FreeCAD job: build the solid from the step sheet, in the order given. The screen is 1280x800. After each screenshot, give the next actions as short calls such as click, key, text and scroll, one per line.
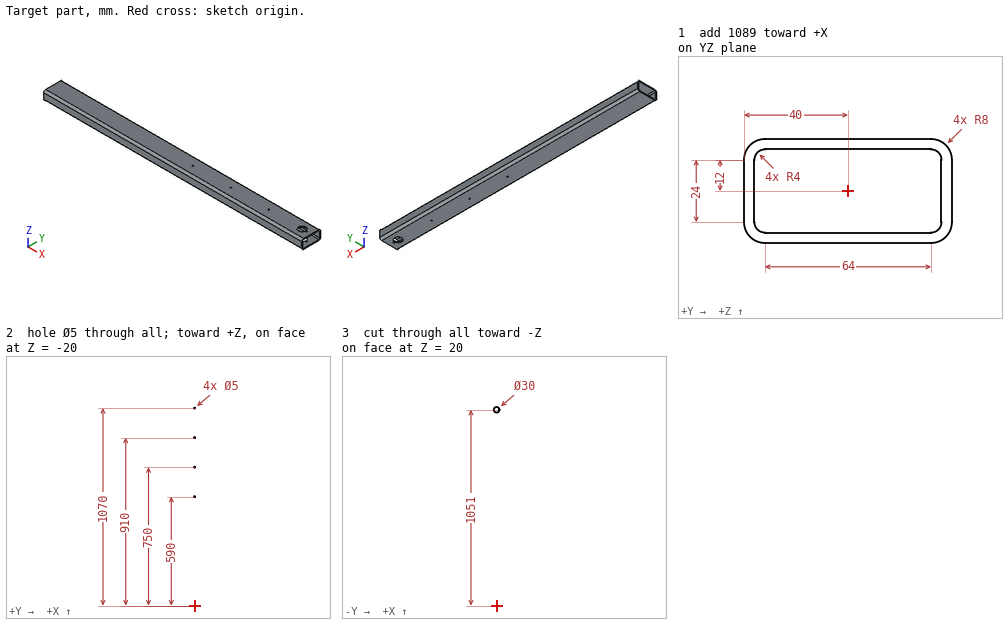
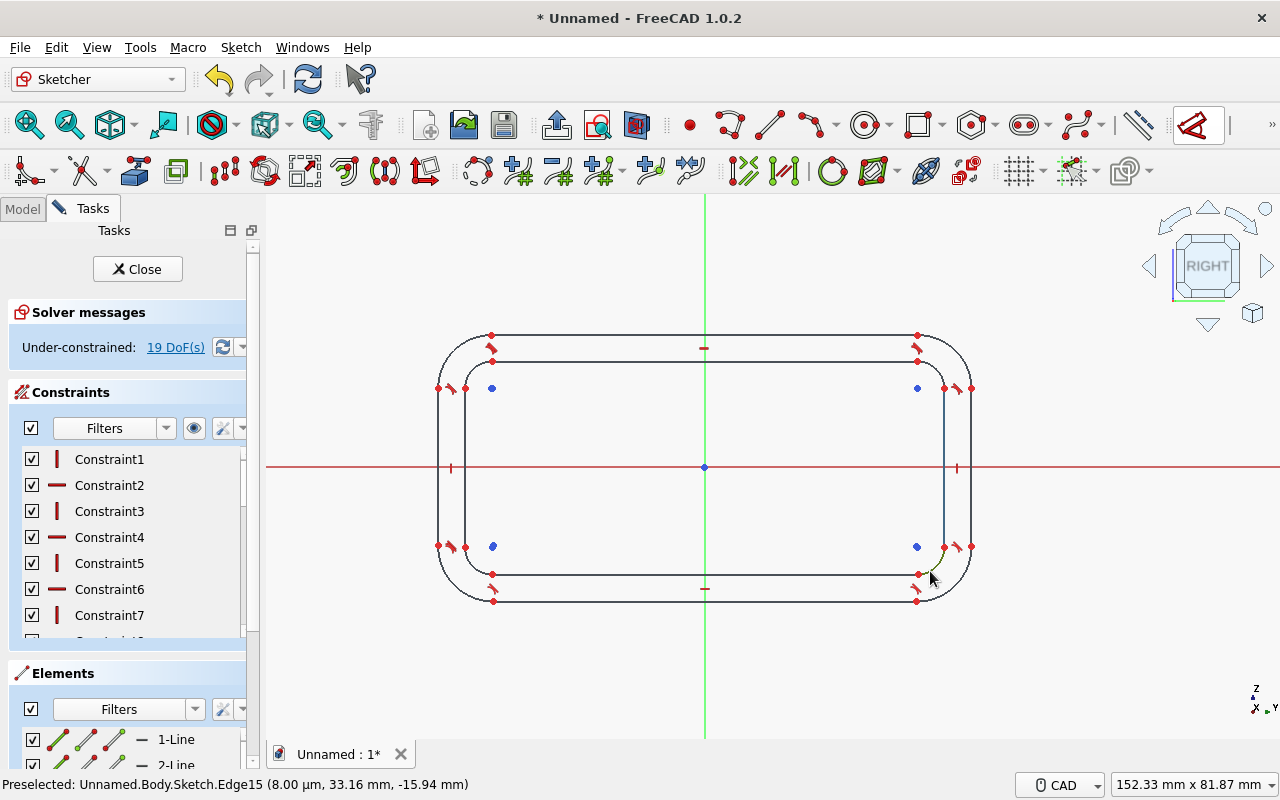
key(t)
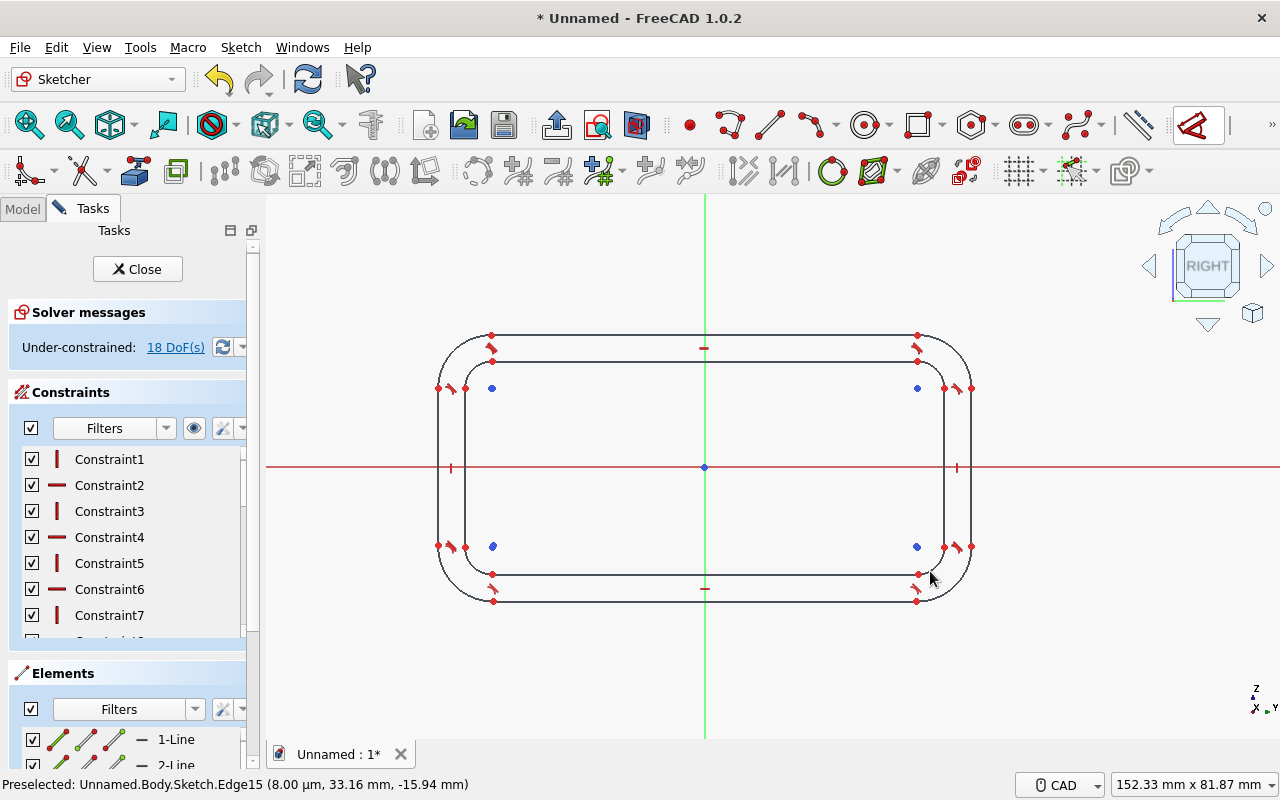
click(790, 575)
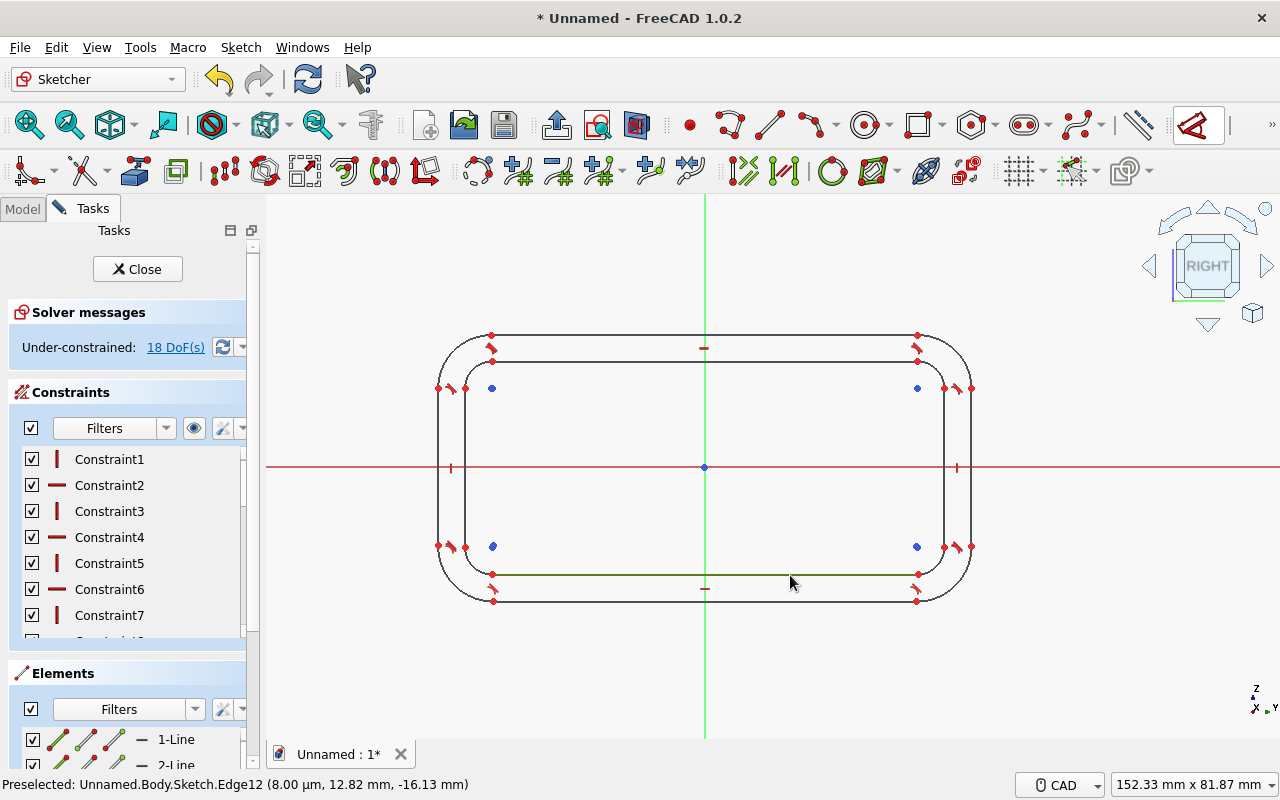
click(930, 571)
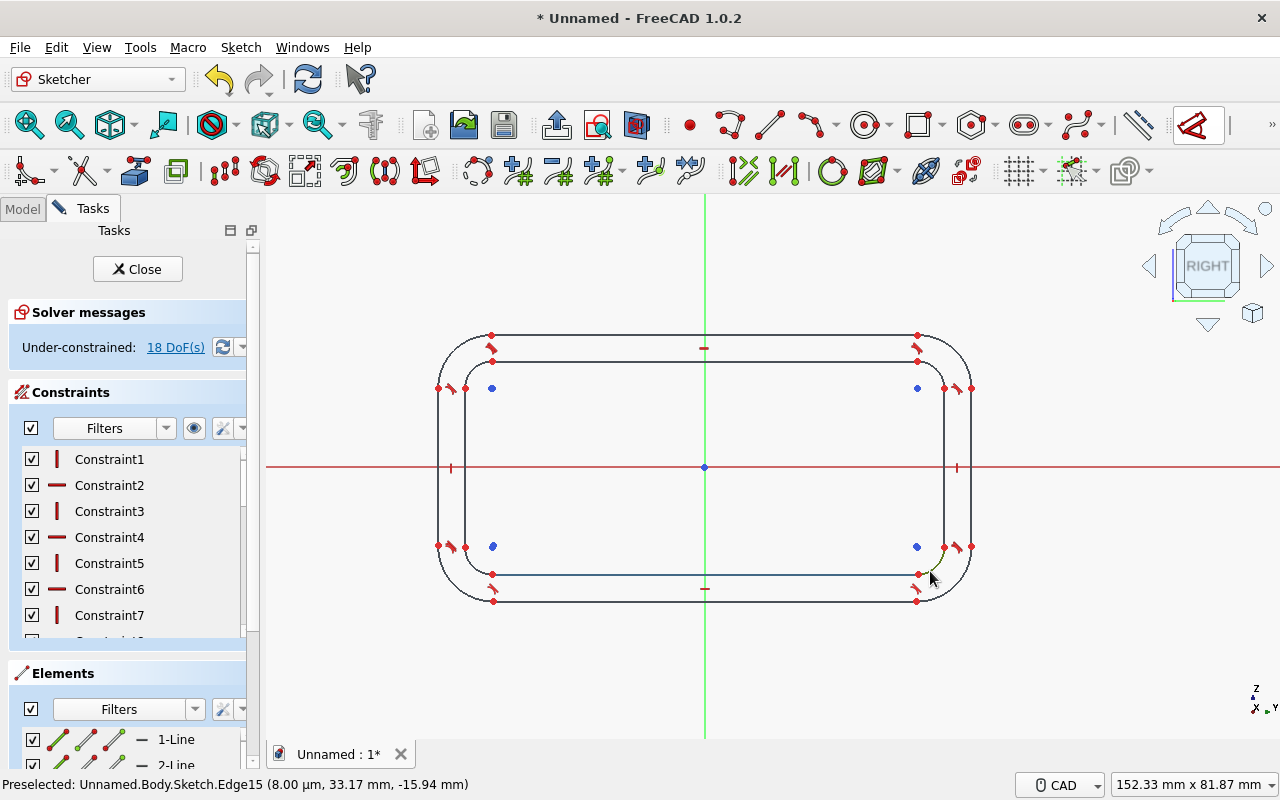
key(t)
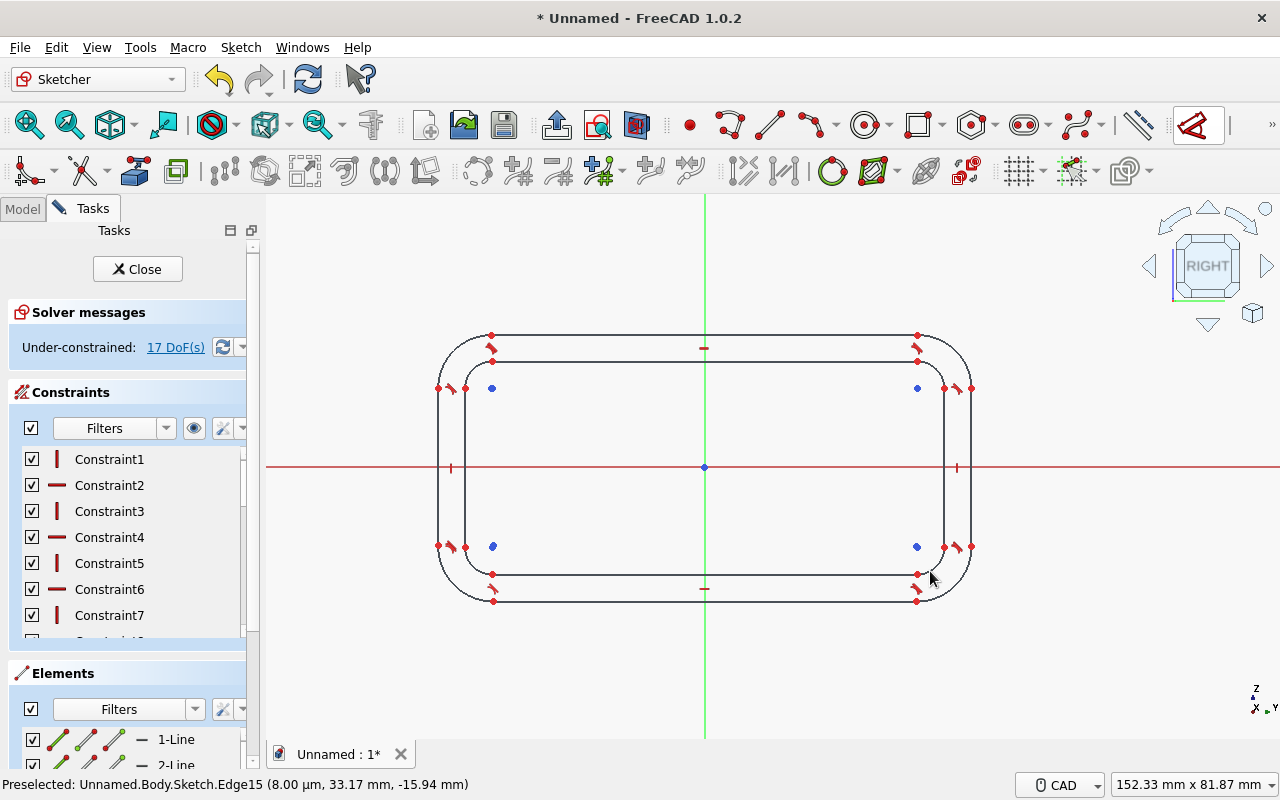
click(790, 575)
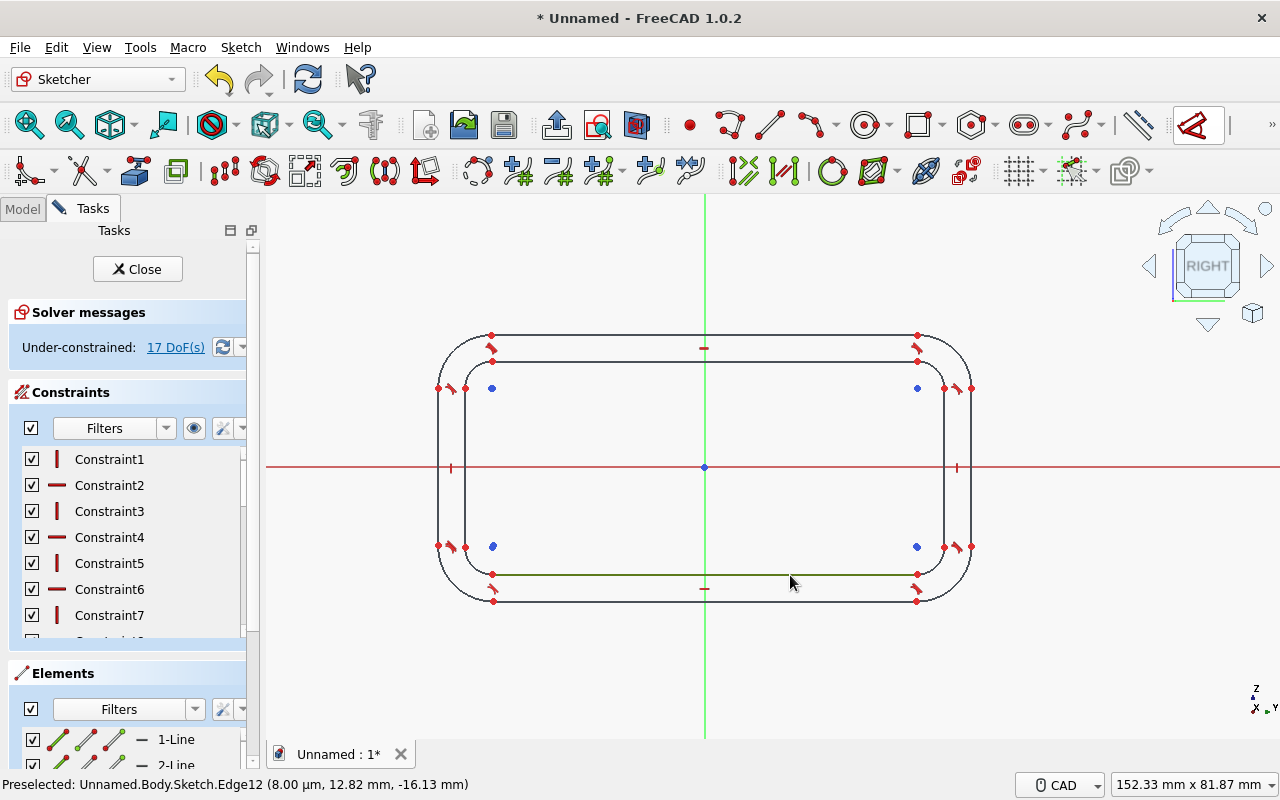
click(468, 560)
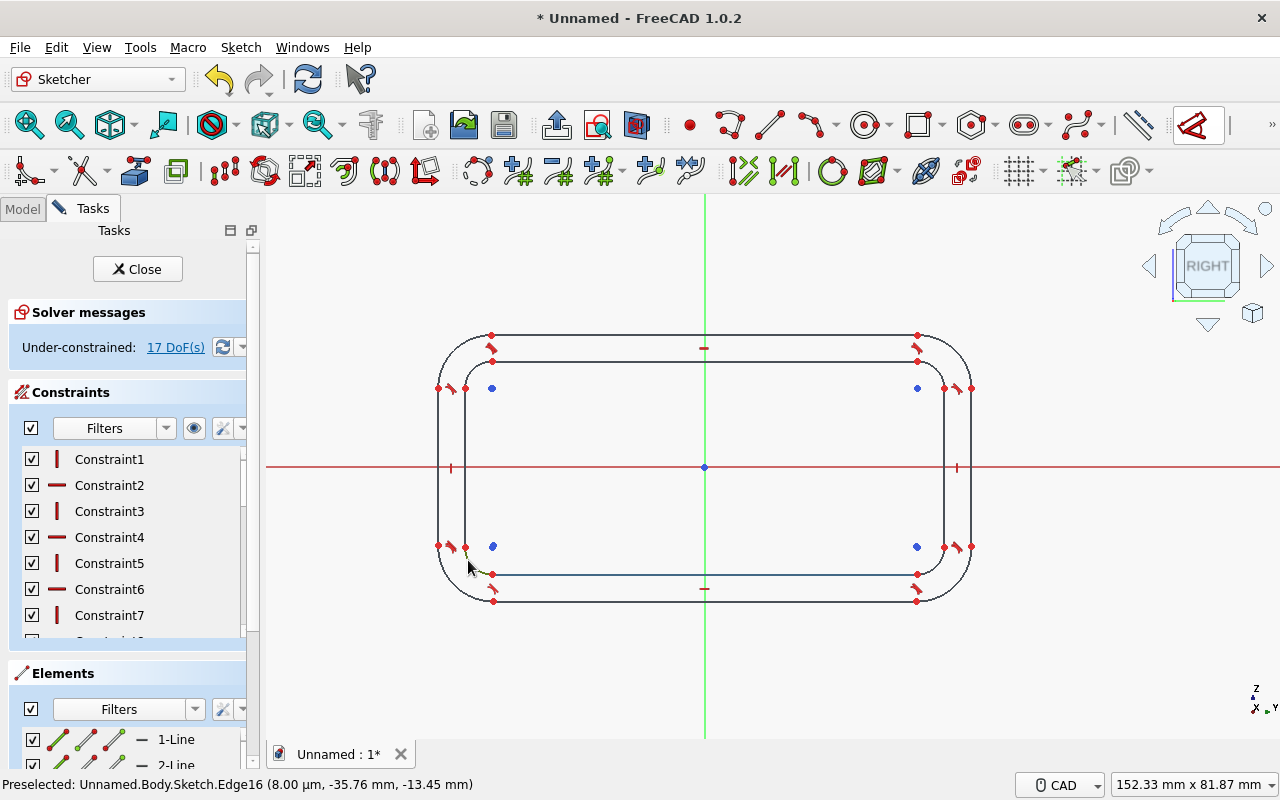
key(t)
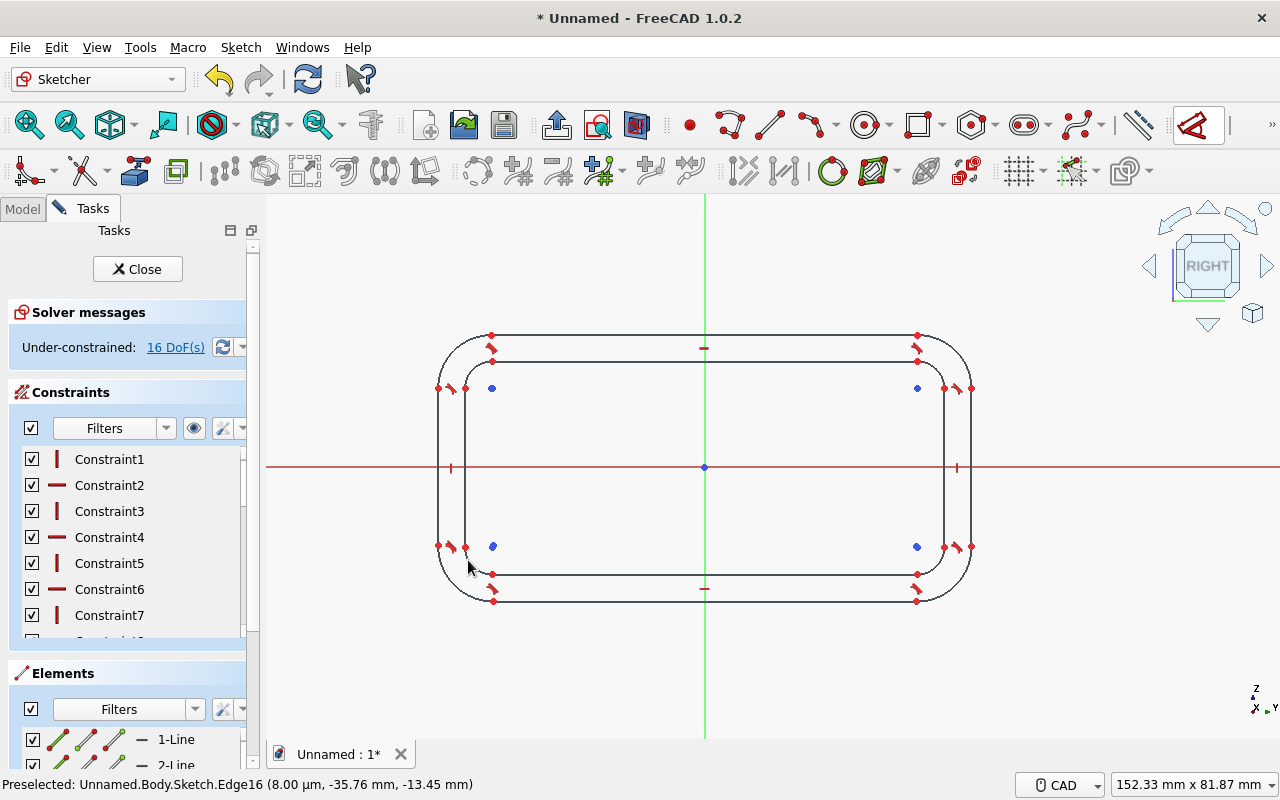
click(467, 341)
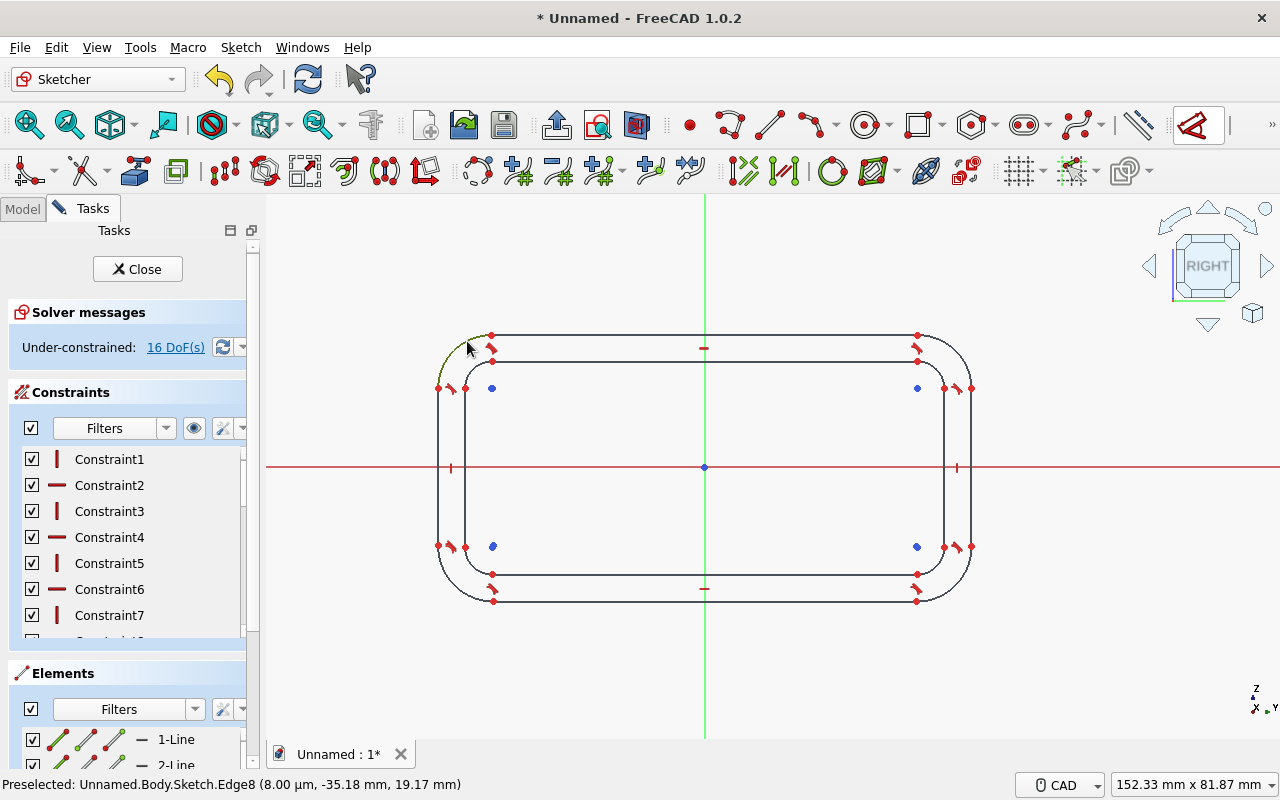
click(480, 364)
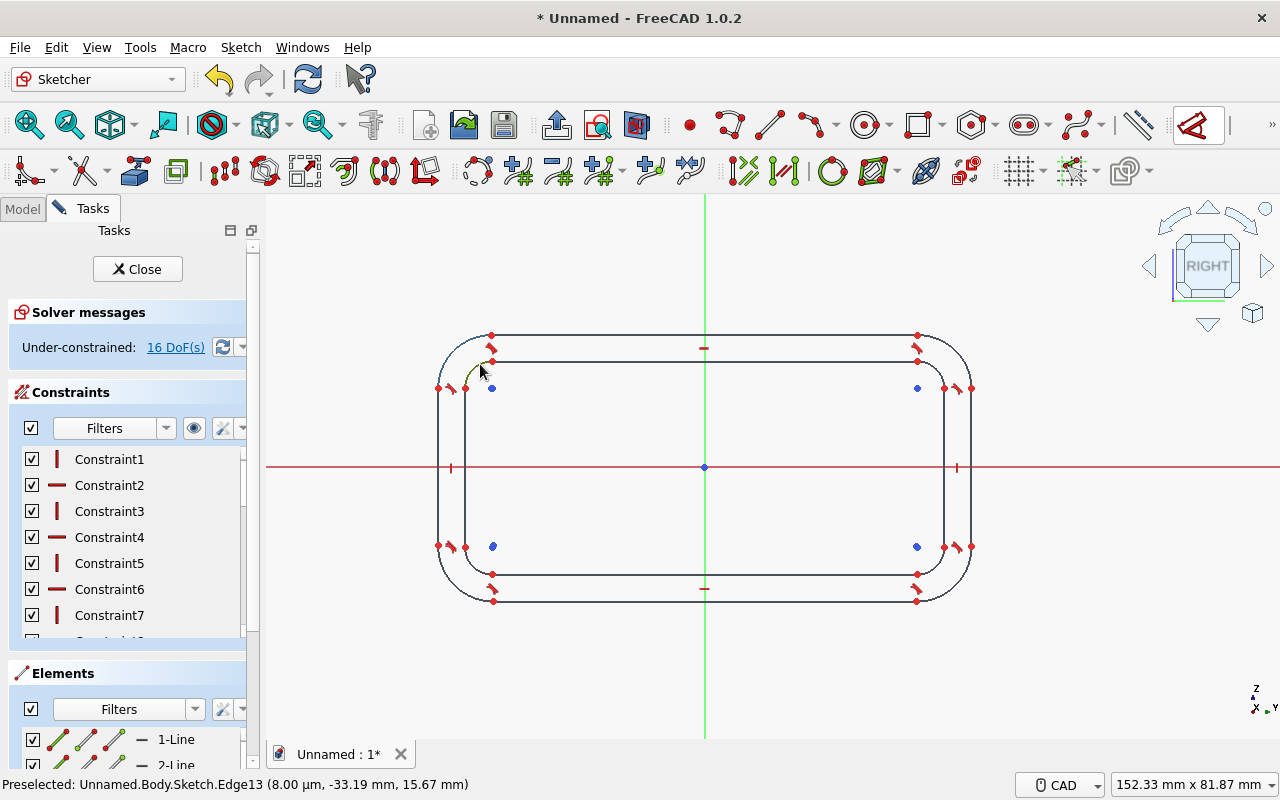
key(c)